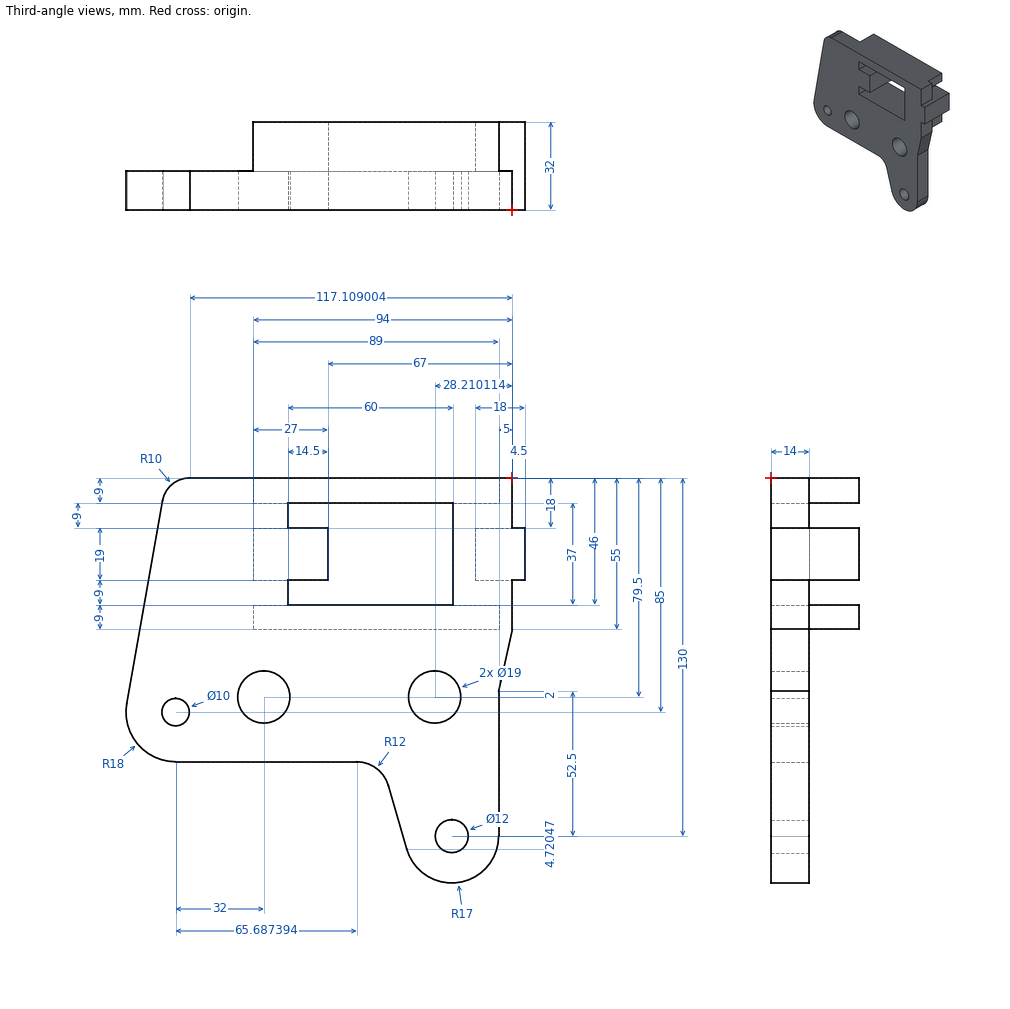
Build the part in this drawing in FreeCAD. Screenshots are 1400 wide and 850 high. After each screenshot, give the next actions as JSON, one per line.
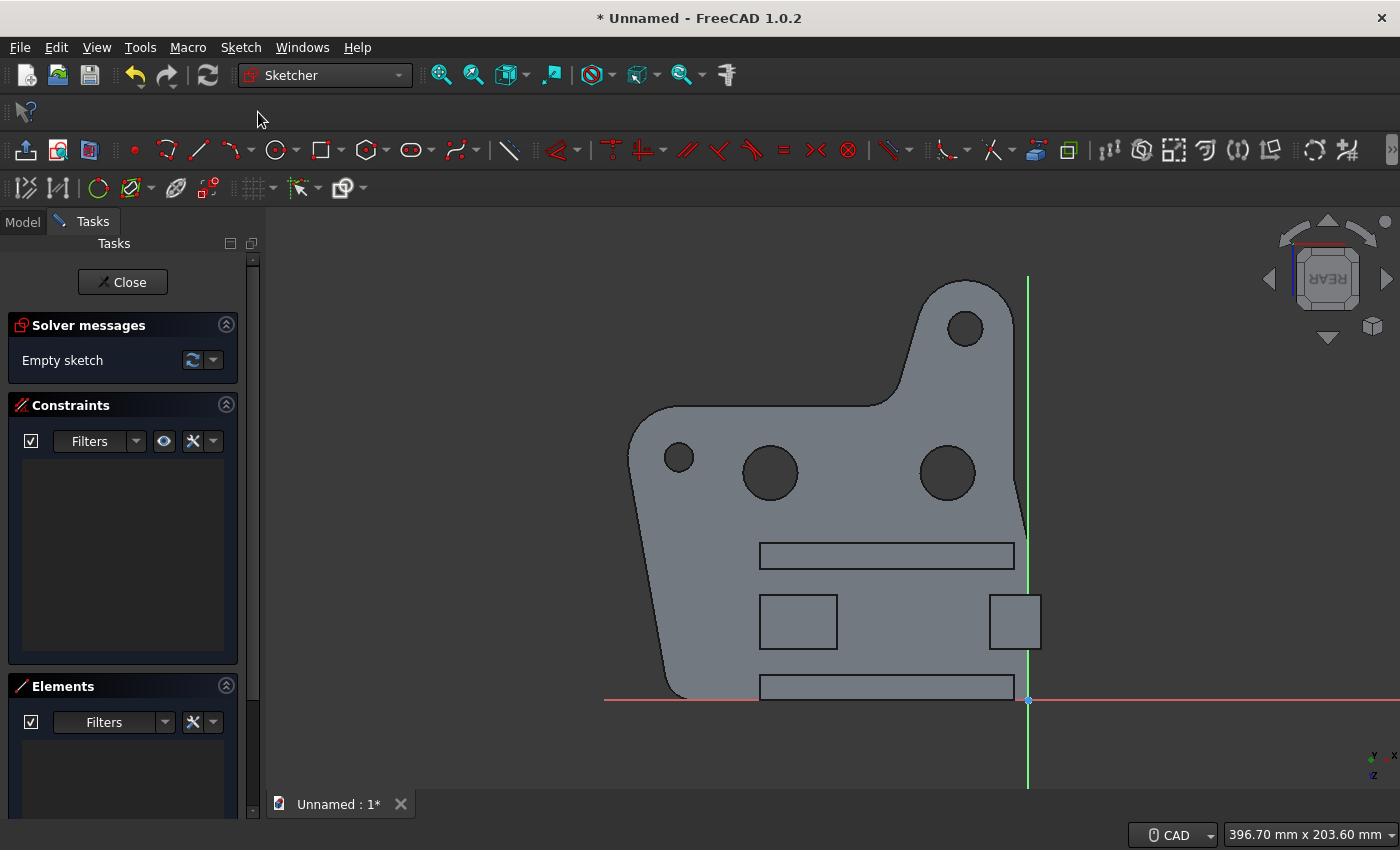
{"action": "scroll", "coordinate": [998, 714], "scroll_direction": "up", "scroll_amount": 5}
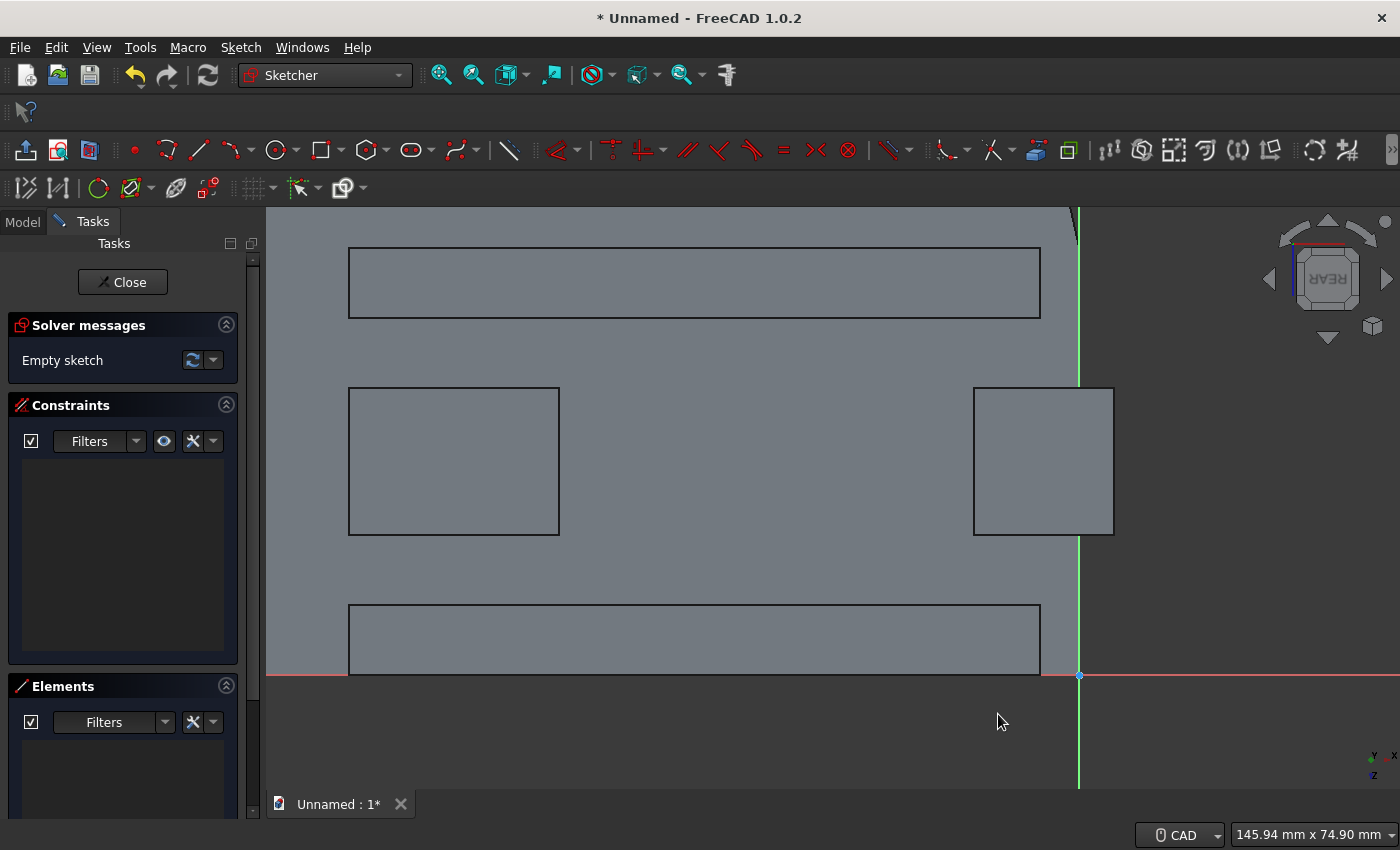
{"action": "left_click", "coordinate": [168, 150]}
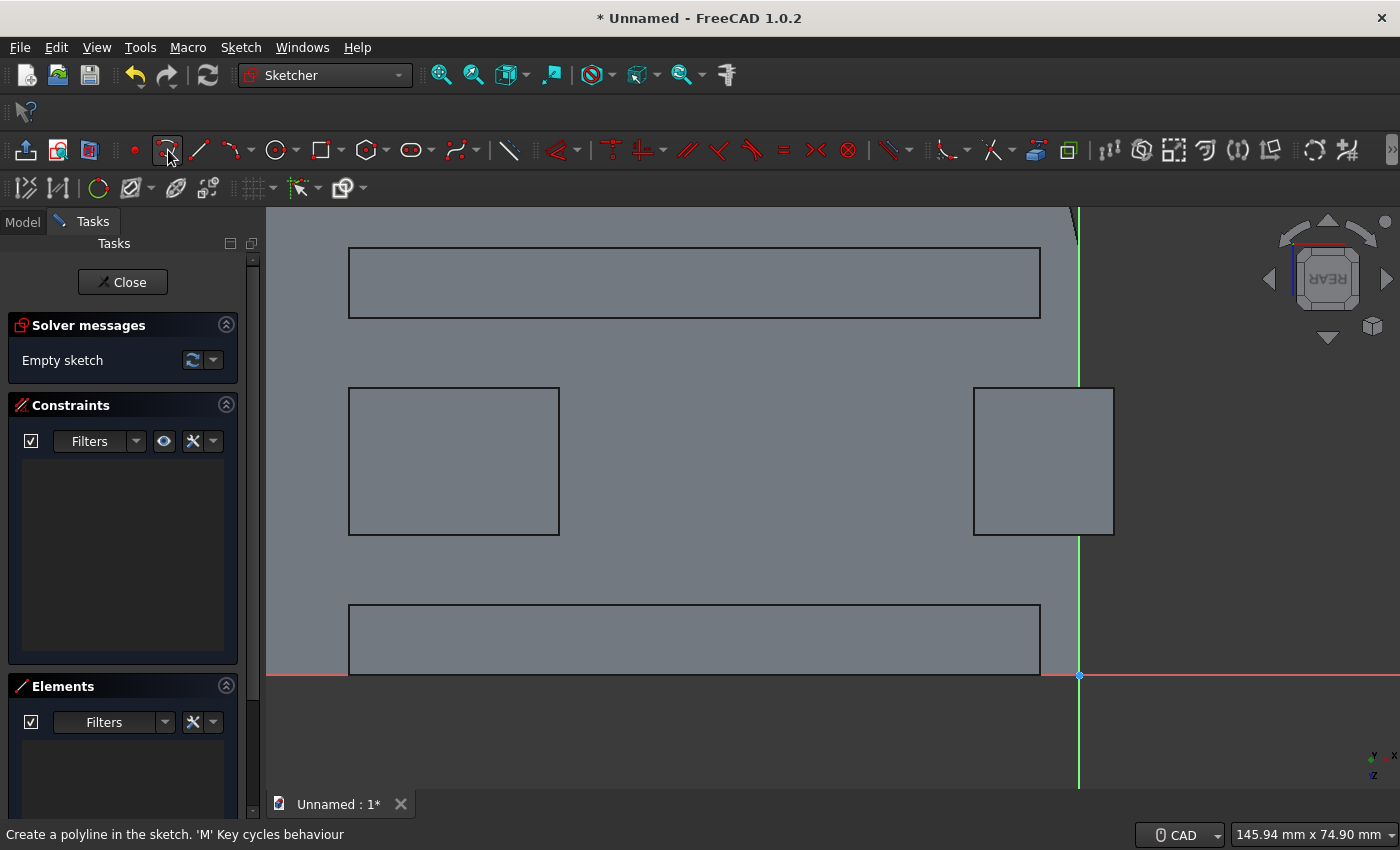
{"action": "left_click", "coordinate": [912, 605]}
{"action": "left_click", "coordinate": [912, 318]}
{"action": "left_click", "coordinate": [446, 318]}
{"action": "left_click", "coordinate": [446, 388]}
{"action": "left_click", "coordinate": [559, 388]}
{"action": "left_click", "coordinate": [559, 535]}
{"action": "left_click", "coordinate": [446, 535]}
{"action": "left_click", "coordinate": [446, 605]}
{"action": "left_click", "coordinate": [912, 606]}
{"action": "key", "text": "Escape"}
{"action": "key", "text": "Escape"}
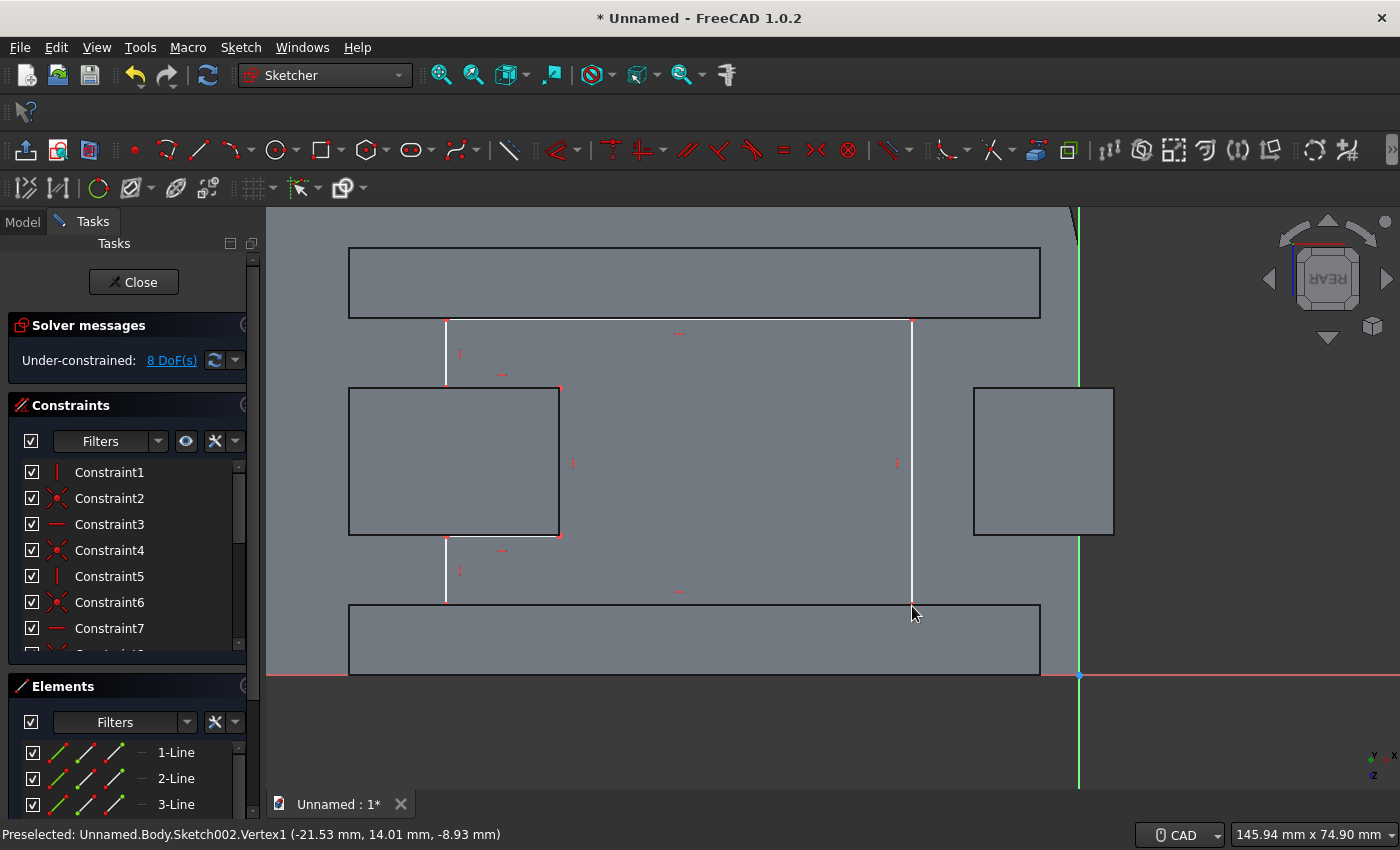
{"action": "left_click", "coordinate": [556, 150]}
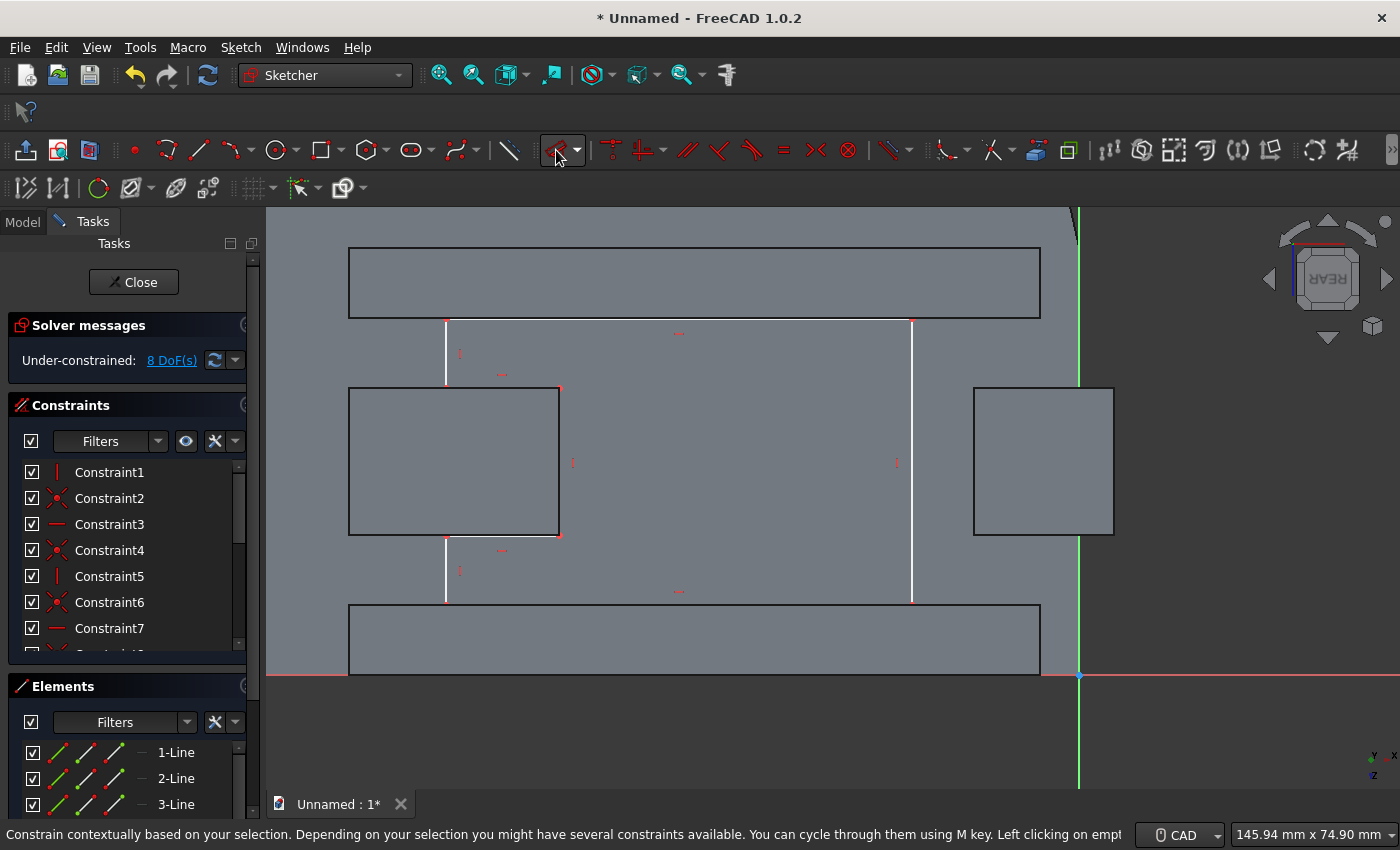
{"action": "left_click", "coordinate": [446, 340]}
{"action": "left_click", "coordinate": [412, 354]}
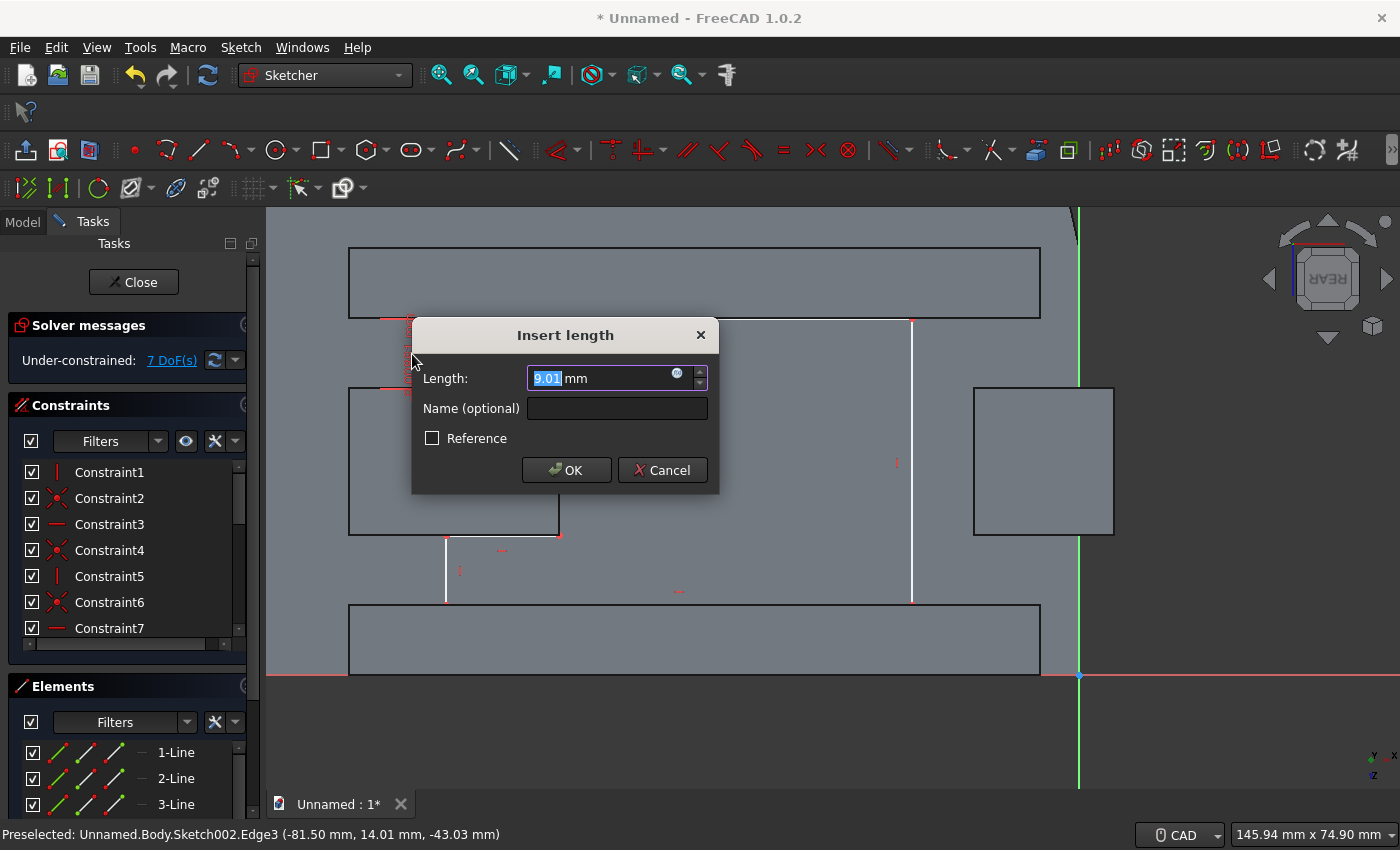
{"action": "type", "text": "9"}
{"action": "key", "text": "Return"}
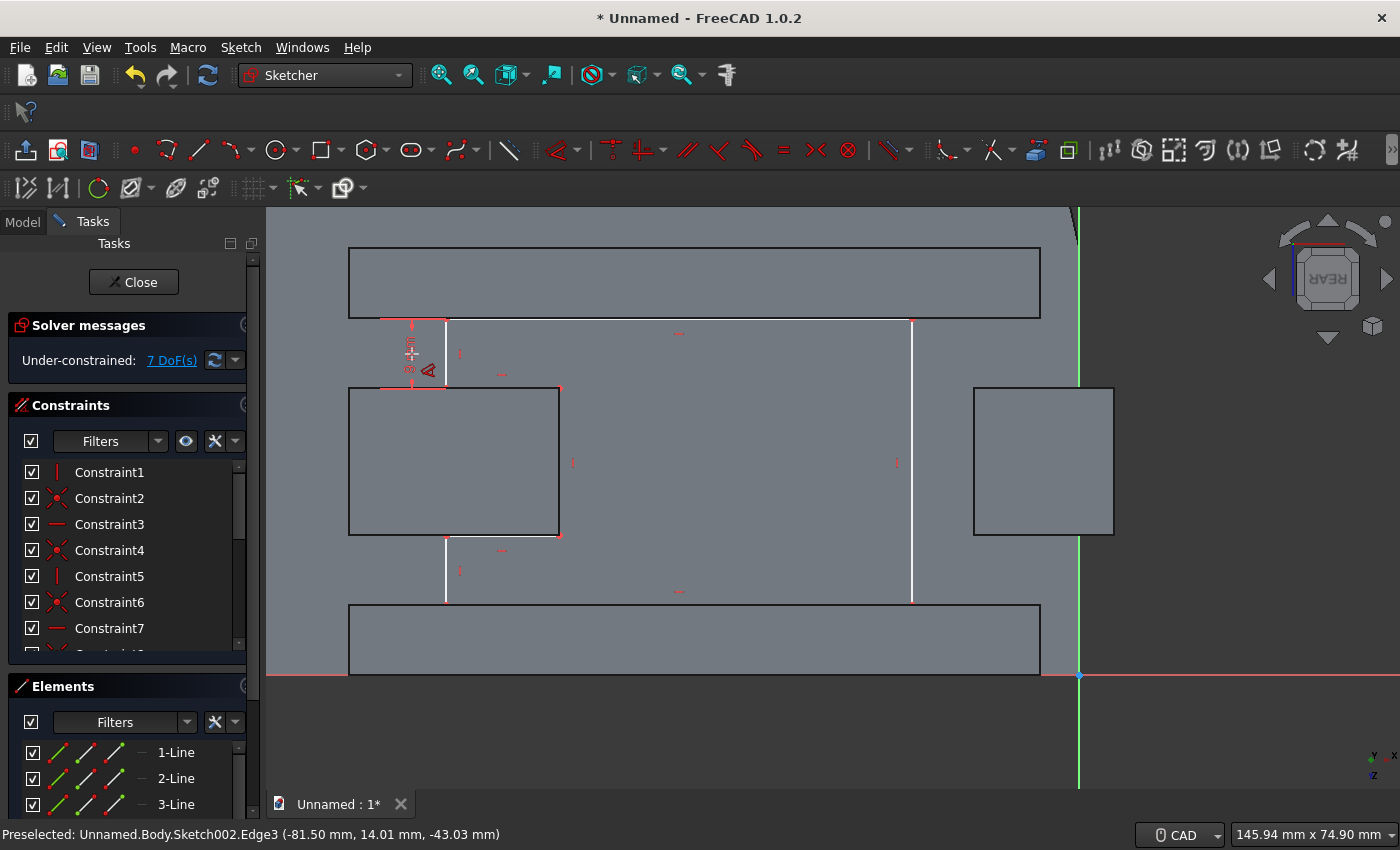
{"action": "left_click", "coordinate": [446, 557]}
{"action": "left_click", "coordinate": [412, 571]}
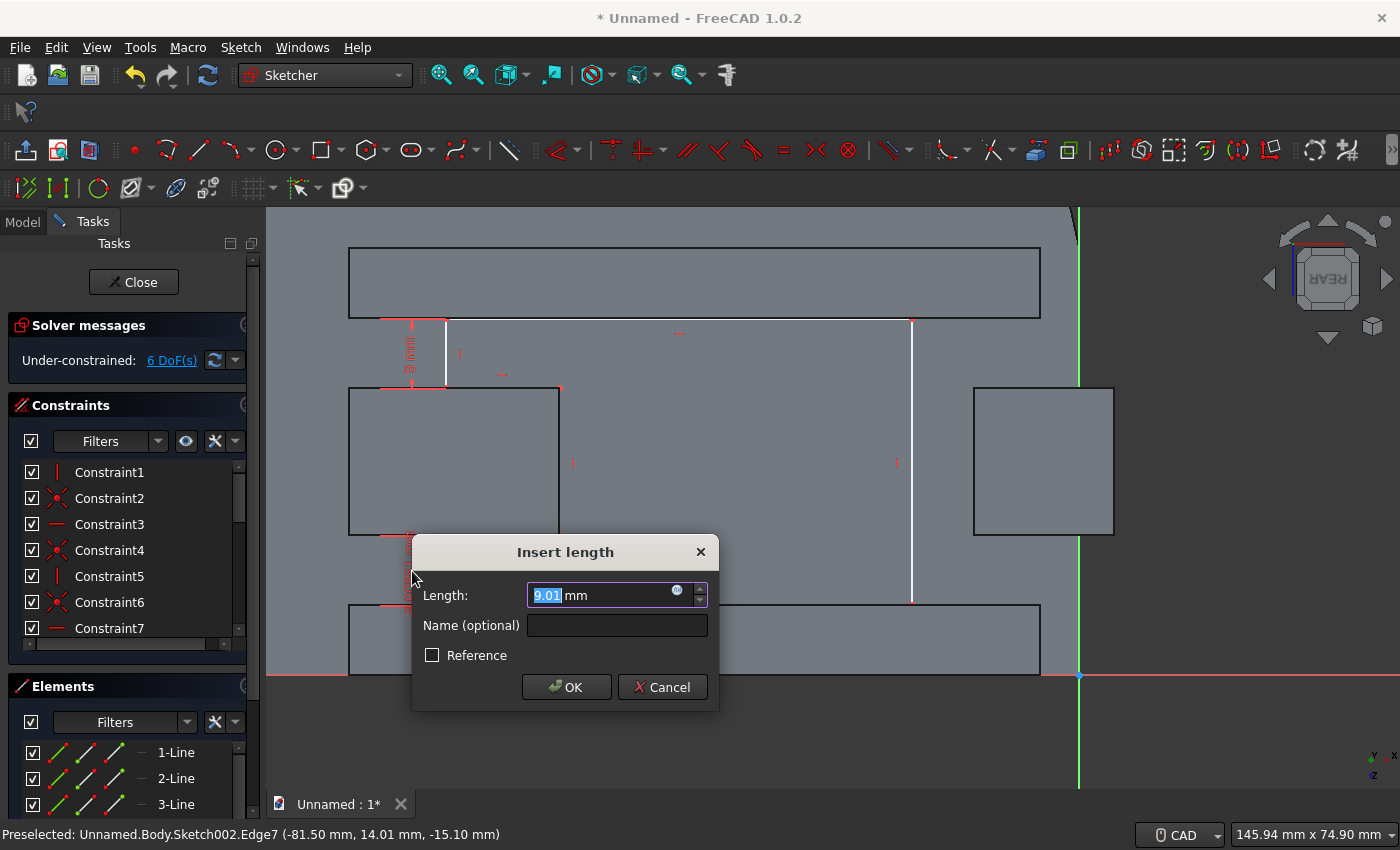
{"action": "type", "text": "9"}
{"action": "key", "text": "Return"}